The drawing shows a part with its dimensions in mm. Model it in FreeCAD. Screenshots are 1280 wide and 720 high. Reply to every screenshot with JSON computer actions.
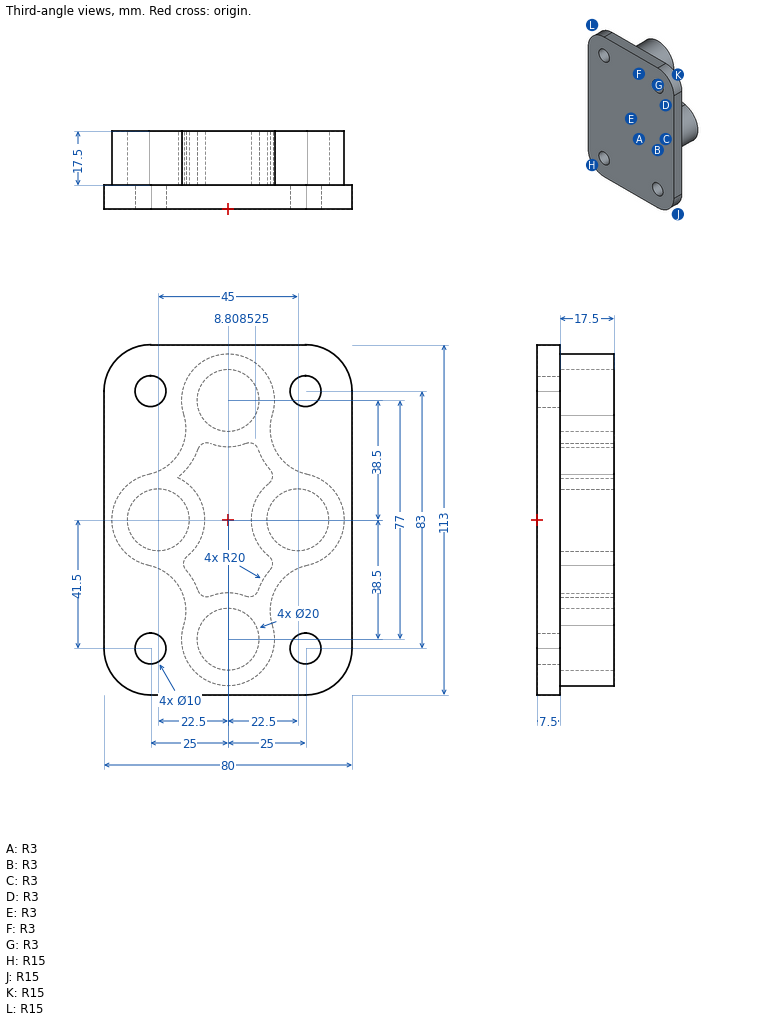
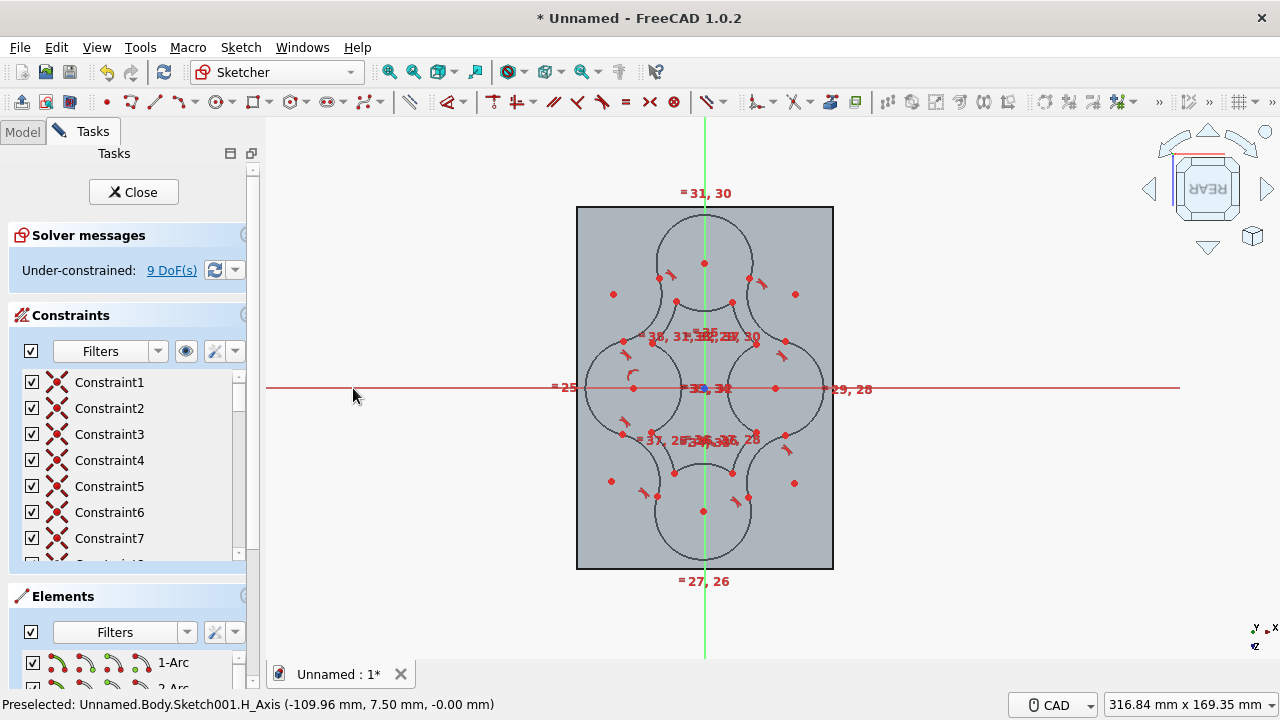
{"action": "left_click", "coordinate": [703, 512]}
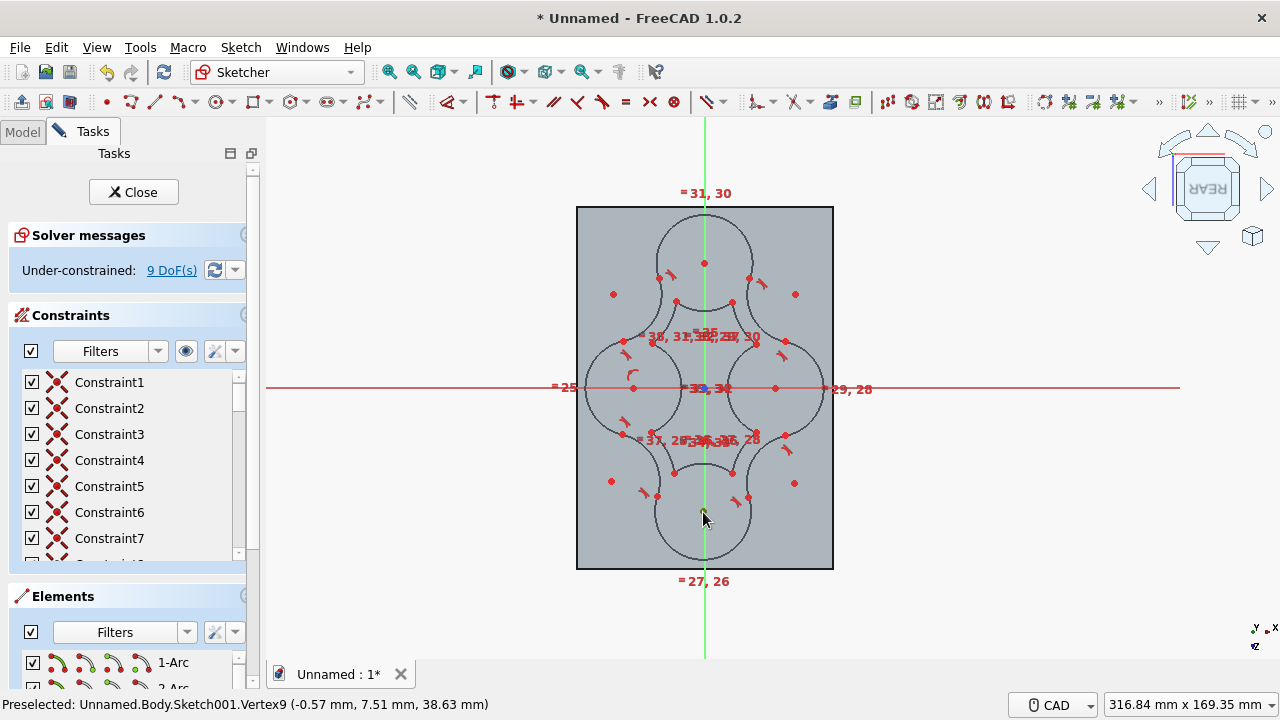
{"action": "left_click", "coordinate": [705, 596]}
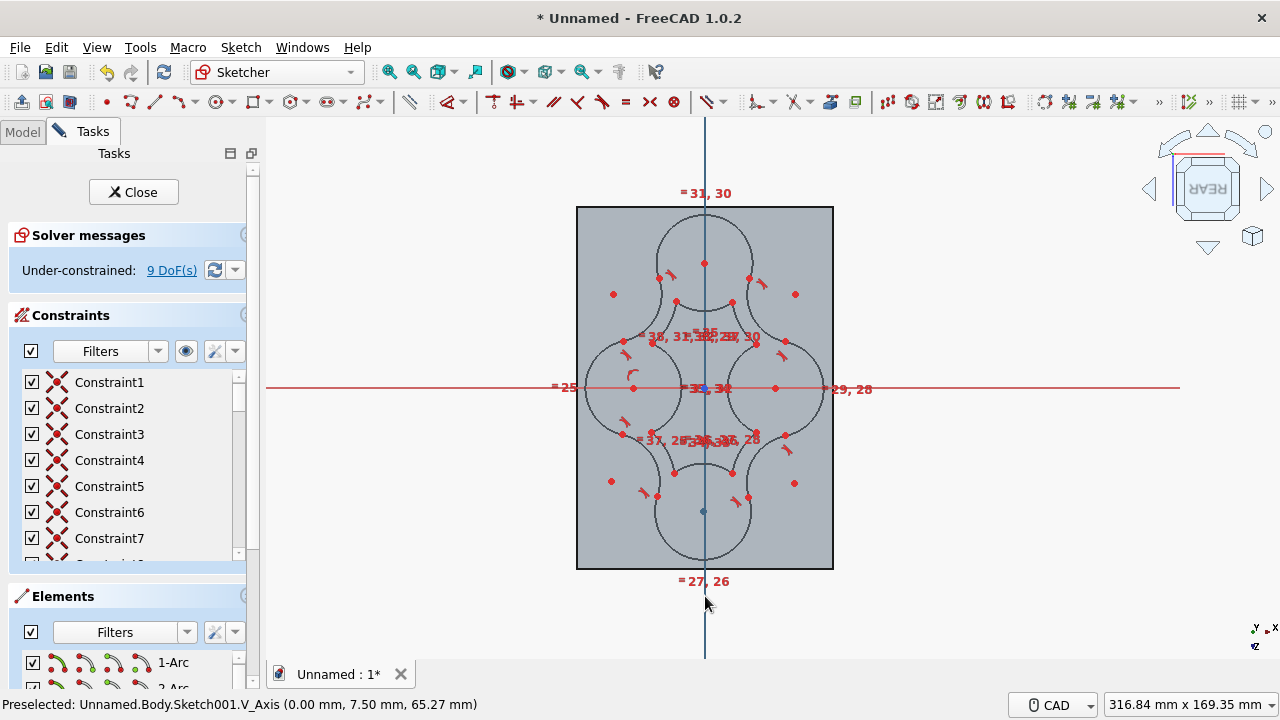
{"action": "left_click", "coordinate": [494, 102]}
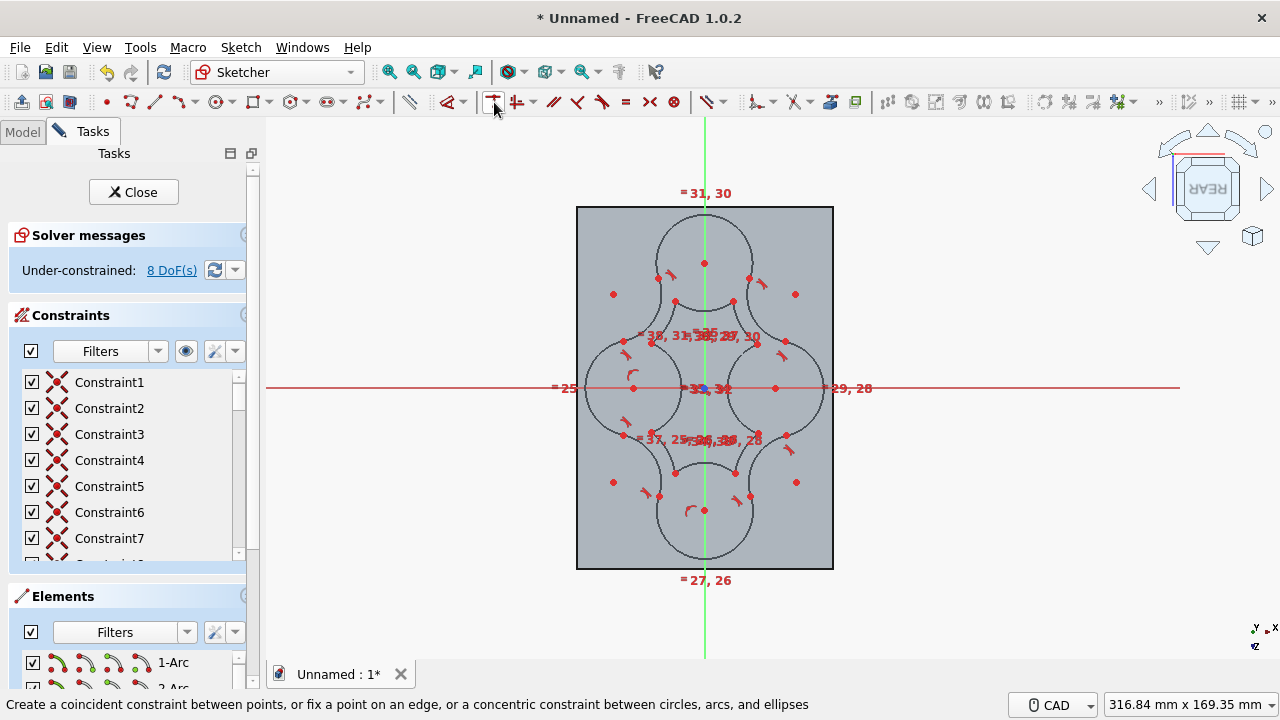
{"action": "left_click", "coordinate": [776, 389]}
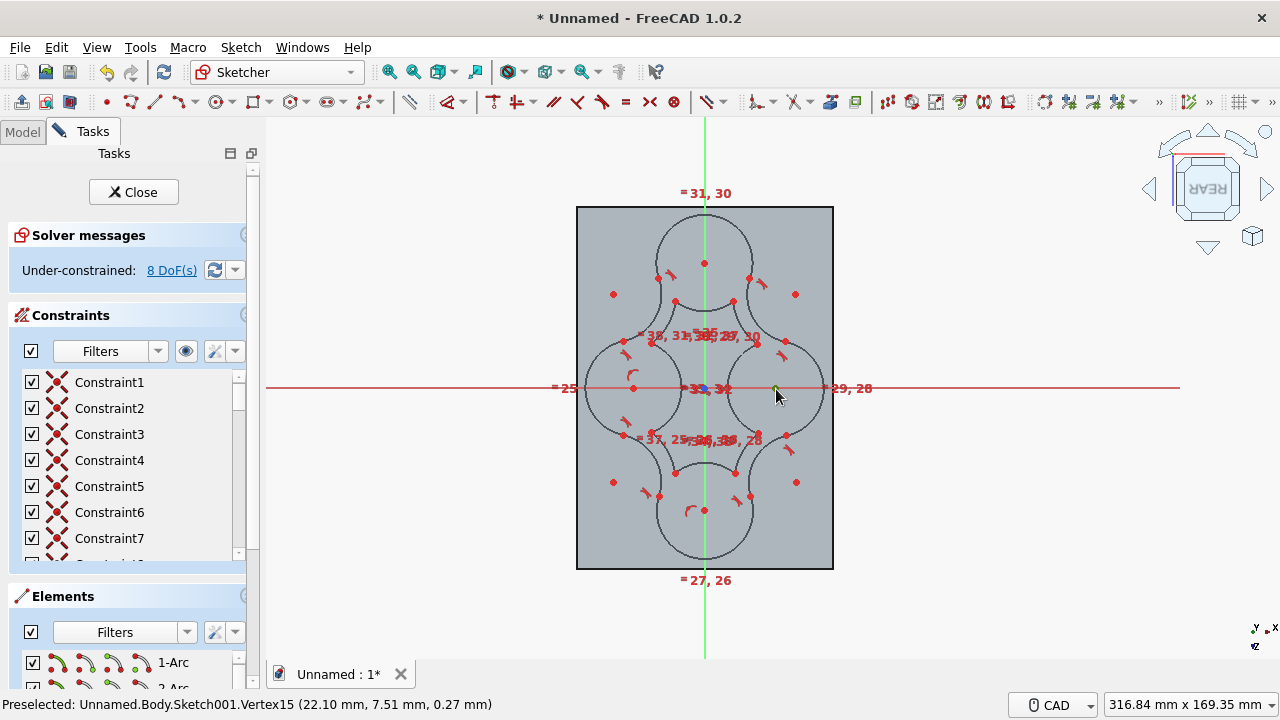
{"action": "left_click", "coordinate": [353, 388]}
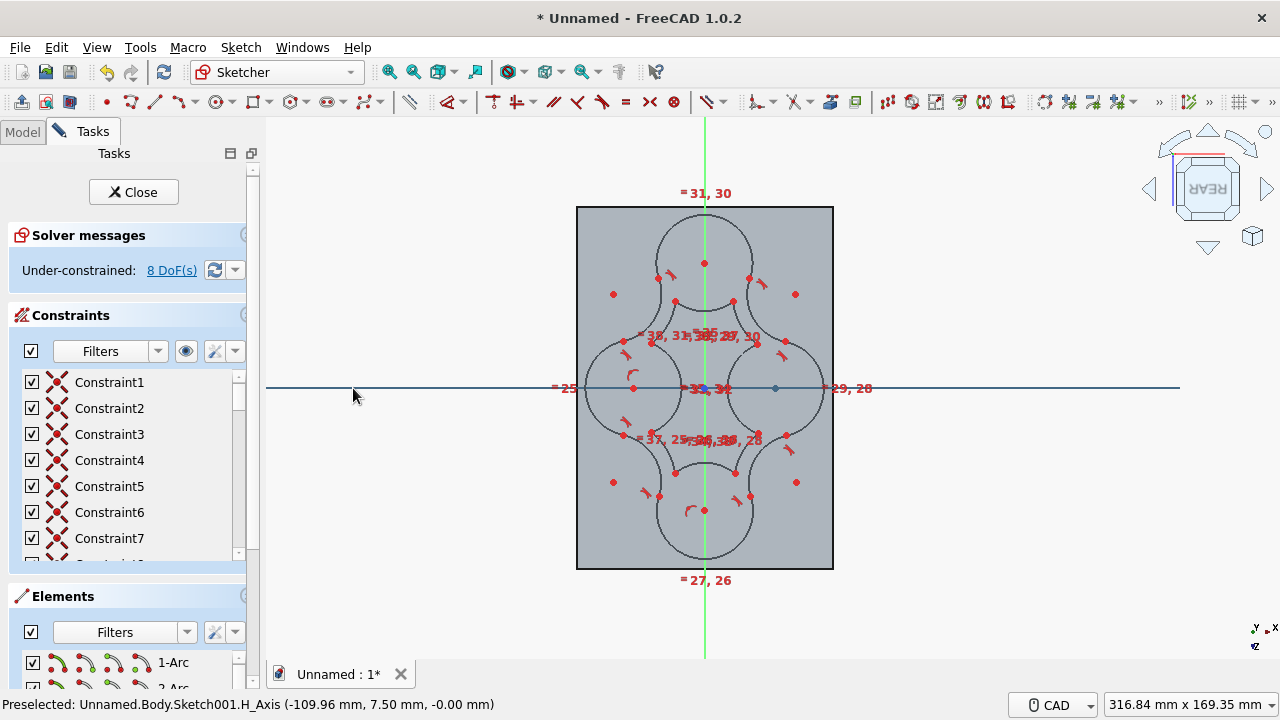
{"action": "key", "text": "c"}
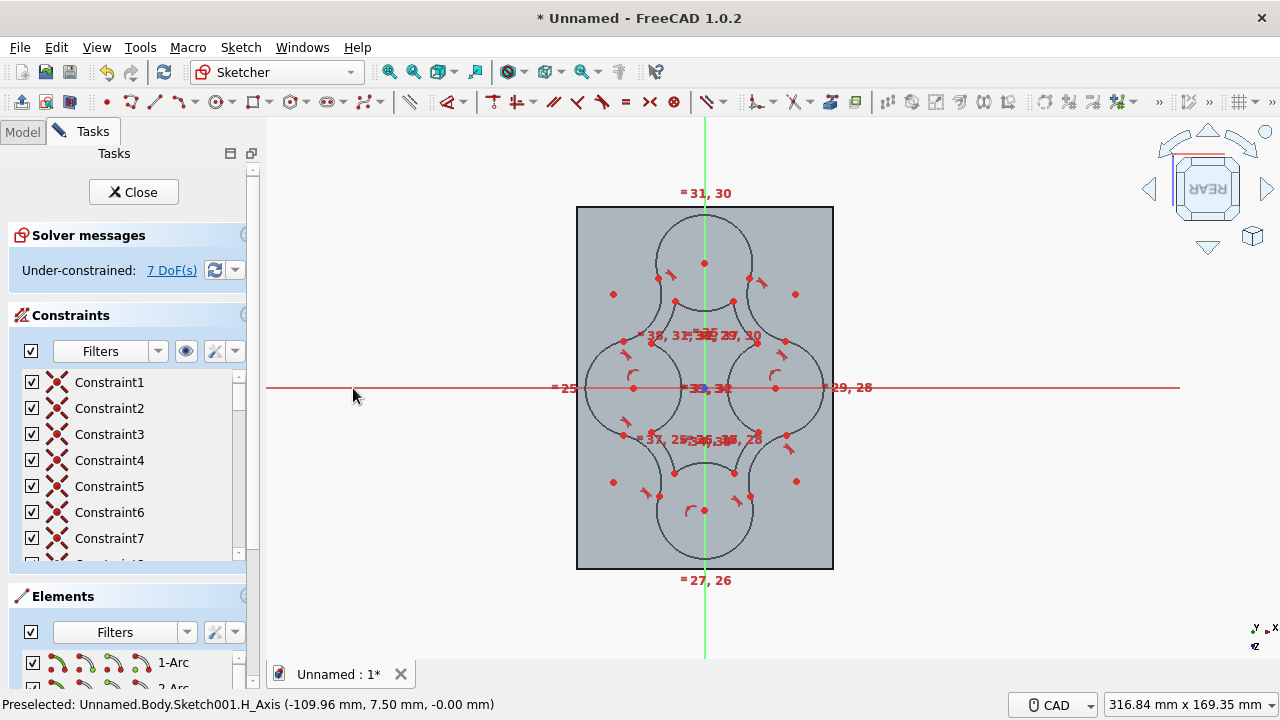
{"action": "left_click", "coordinate": [704, 263]}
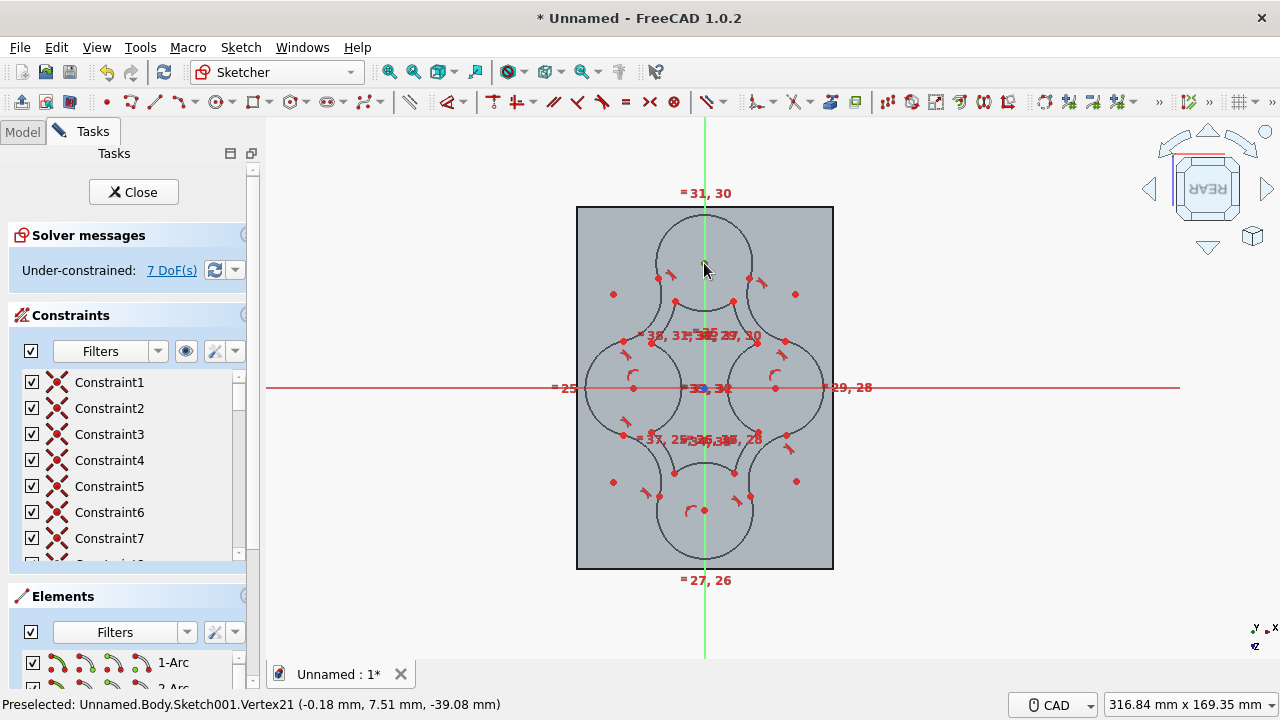
{"action": "left_click", "coordinate": [705, 596]}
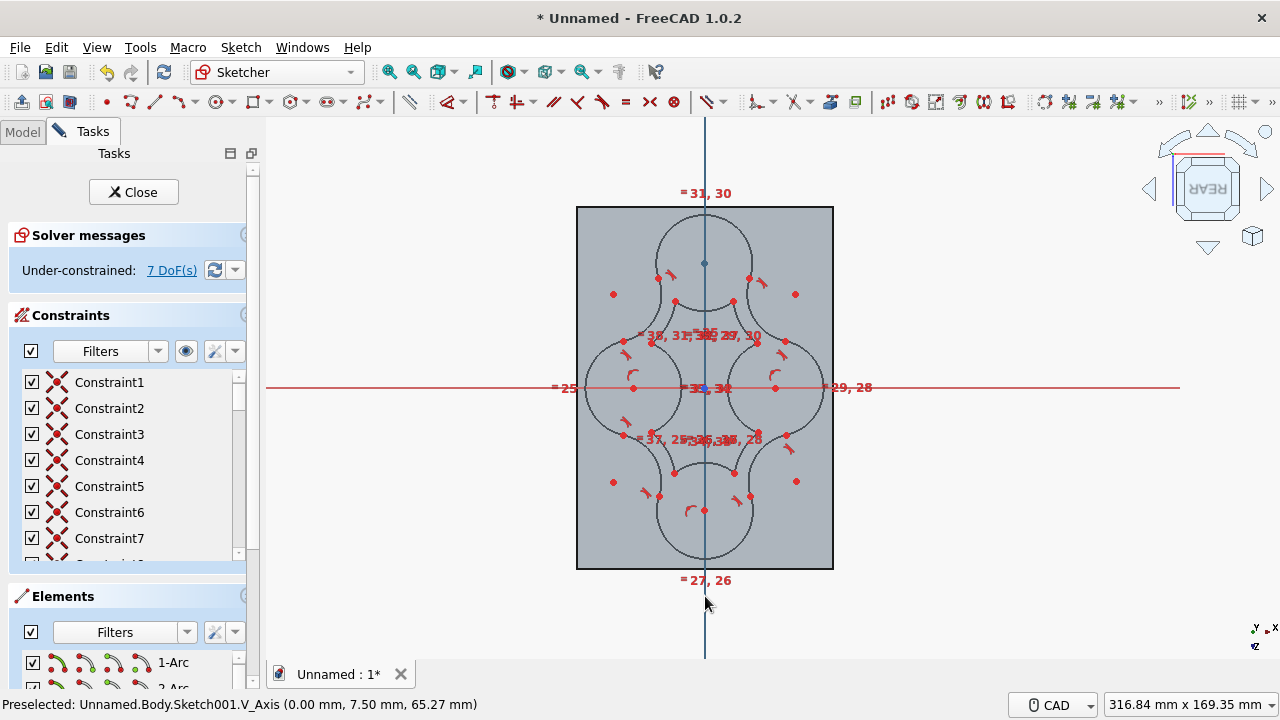
{"action": "left_click", "coordinate": [494, 102]}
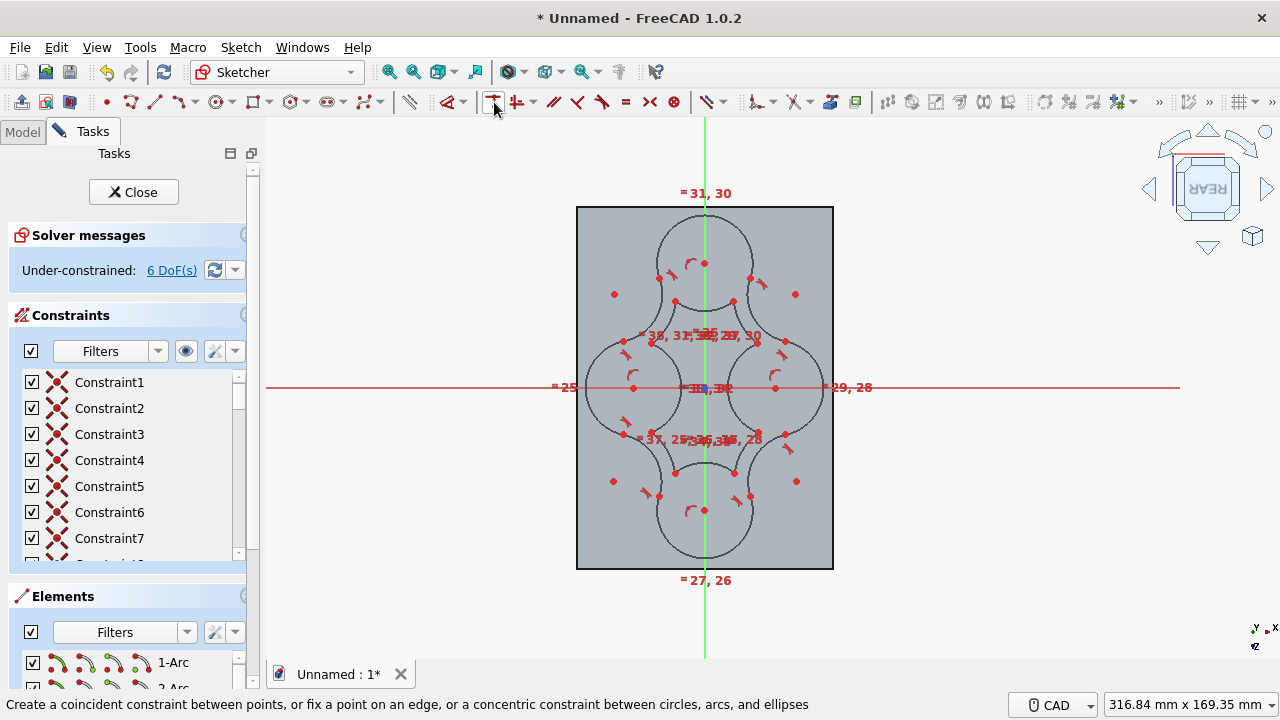
{"action": "key", "text": "d"}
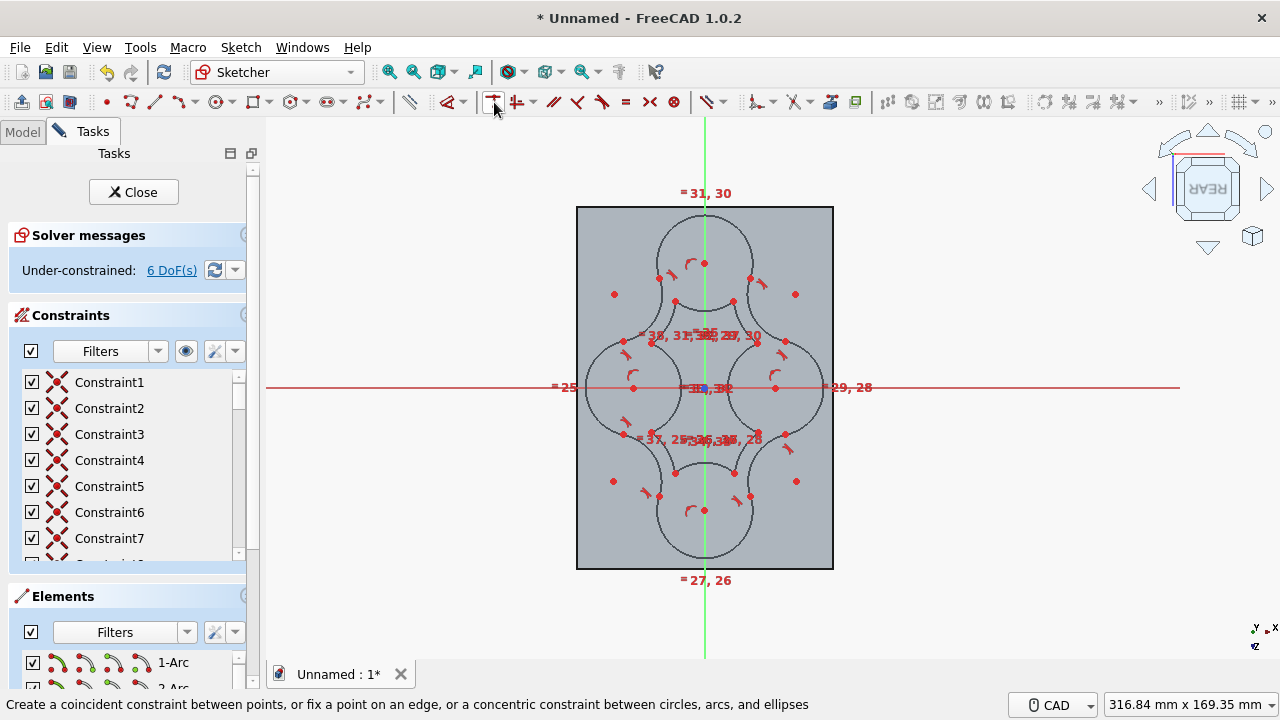
{"action": "left_click", "coordinate": [748, 443]}
{"action": "left_click", "coordinate": [723, 423]}